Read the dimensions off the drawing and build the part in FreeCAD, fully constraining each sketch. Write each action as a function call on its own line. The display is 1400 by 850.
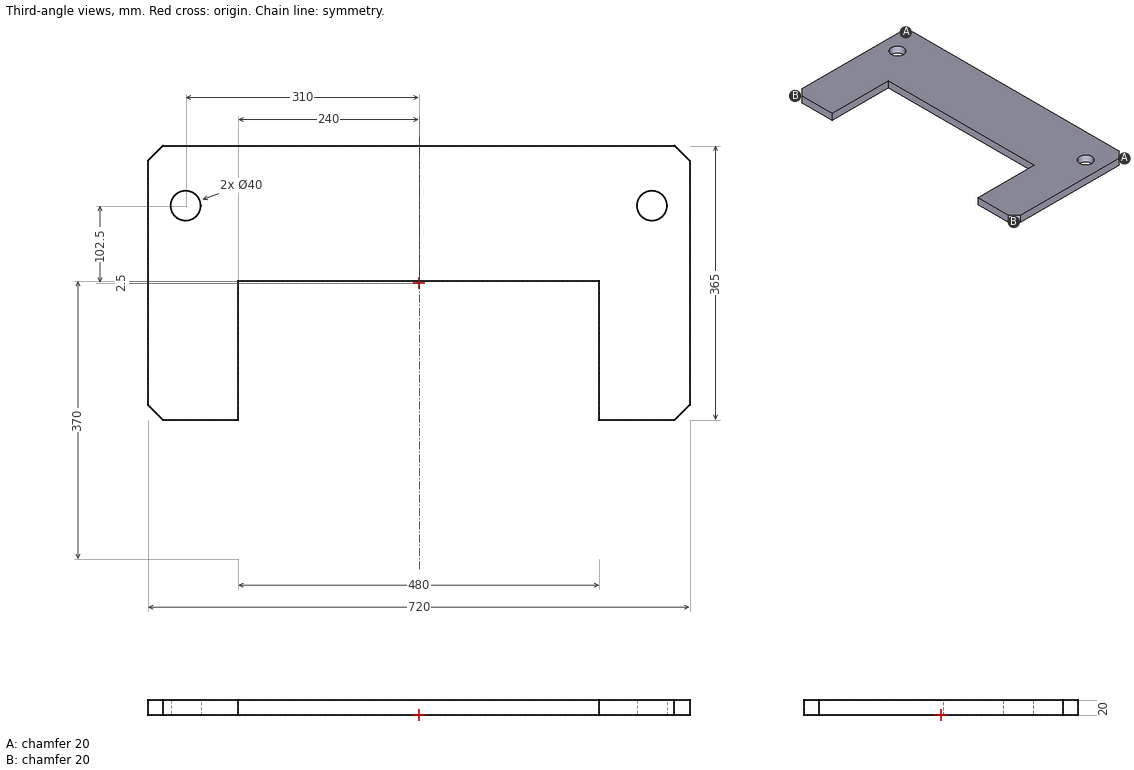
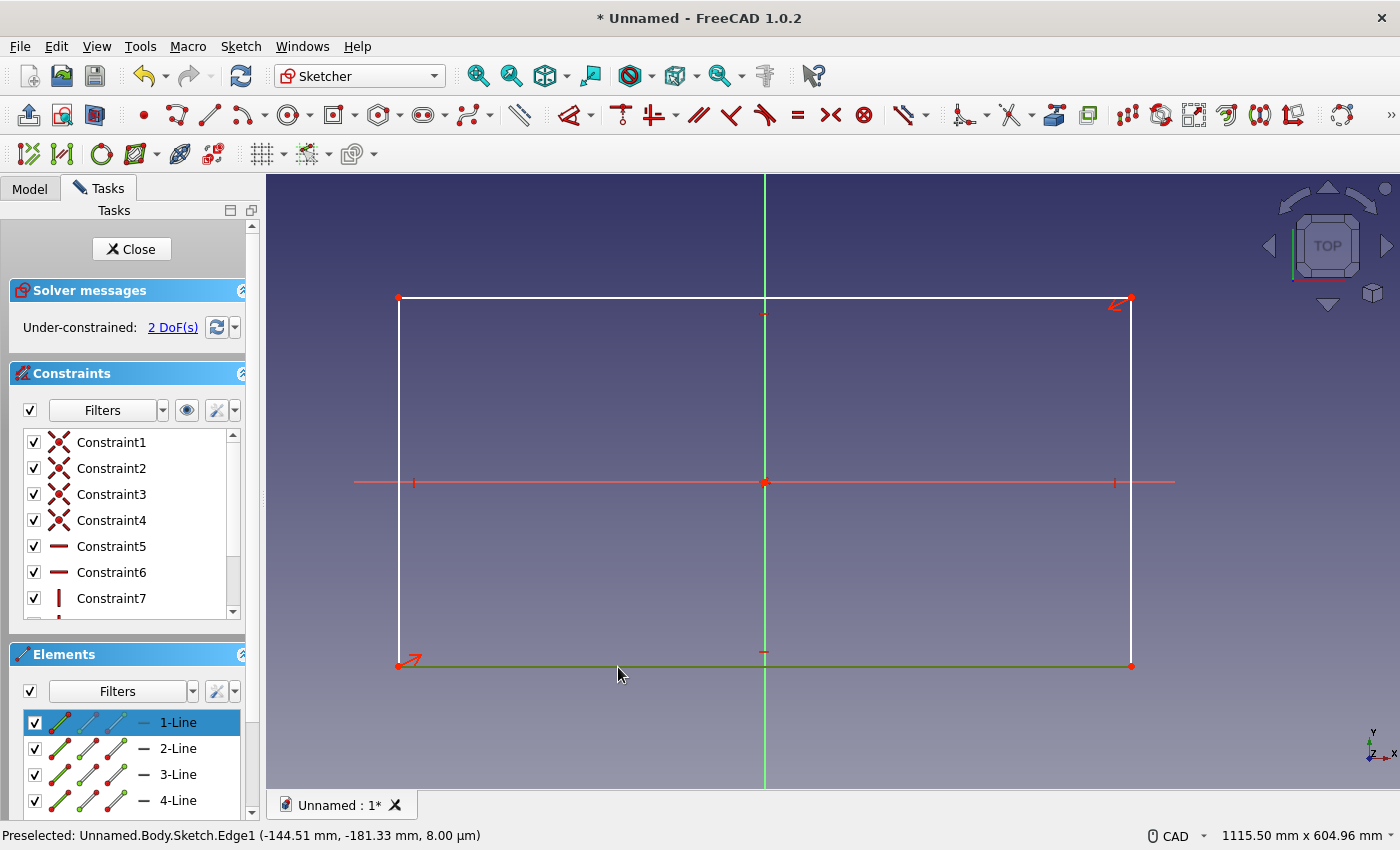
click(590, 116)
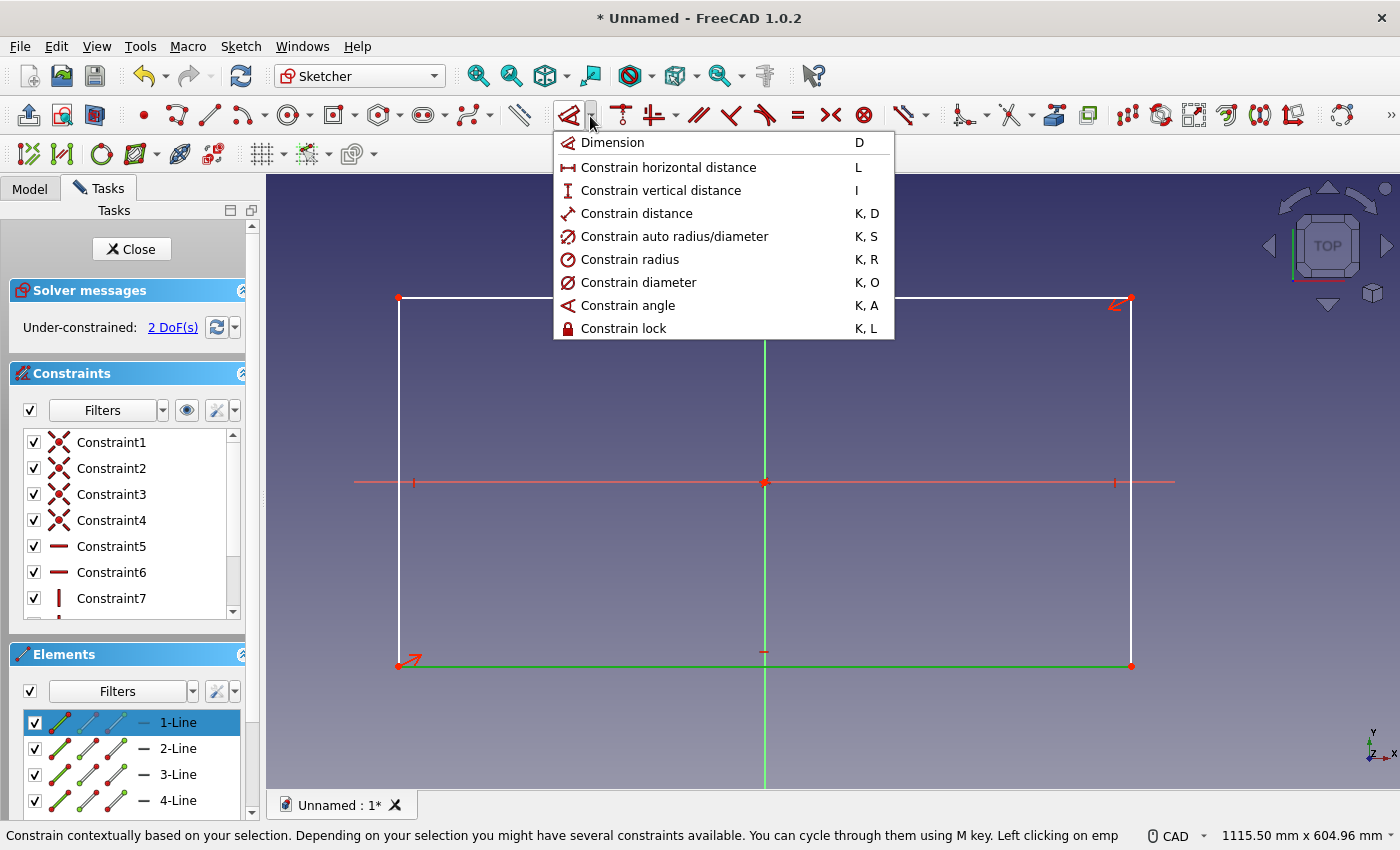
click(724, 168)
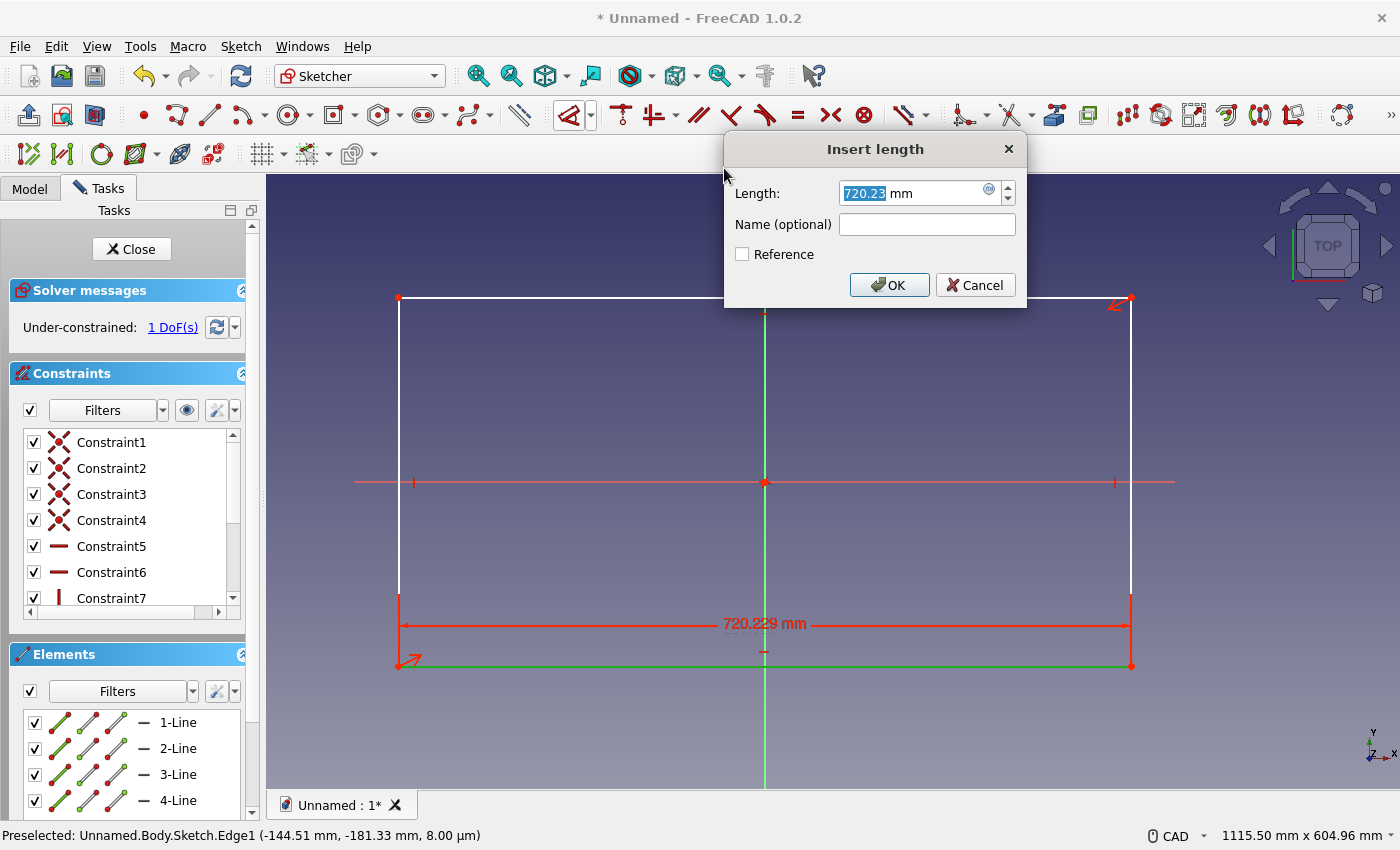
text(720)
key(Return)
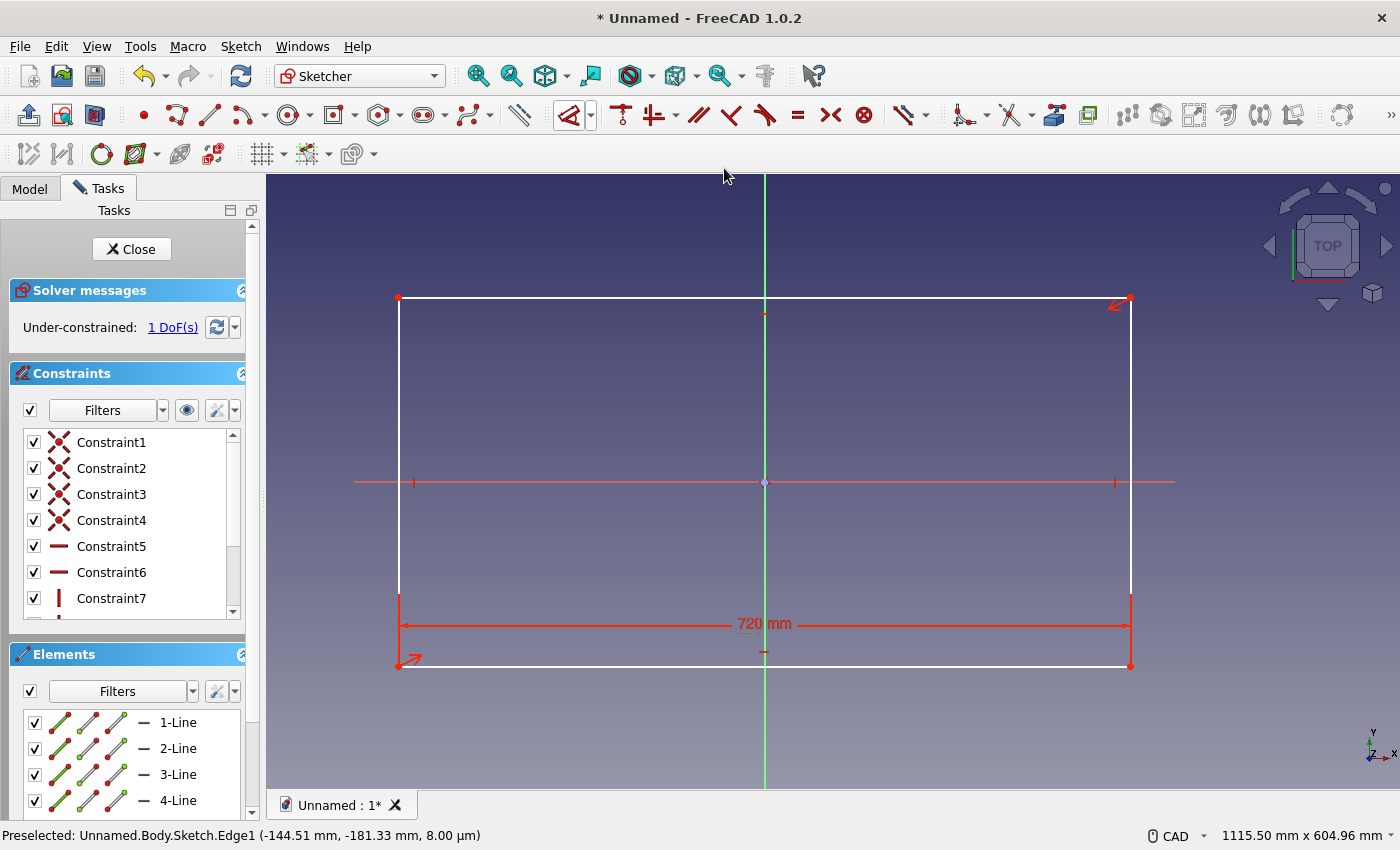
click(1131, 556)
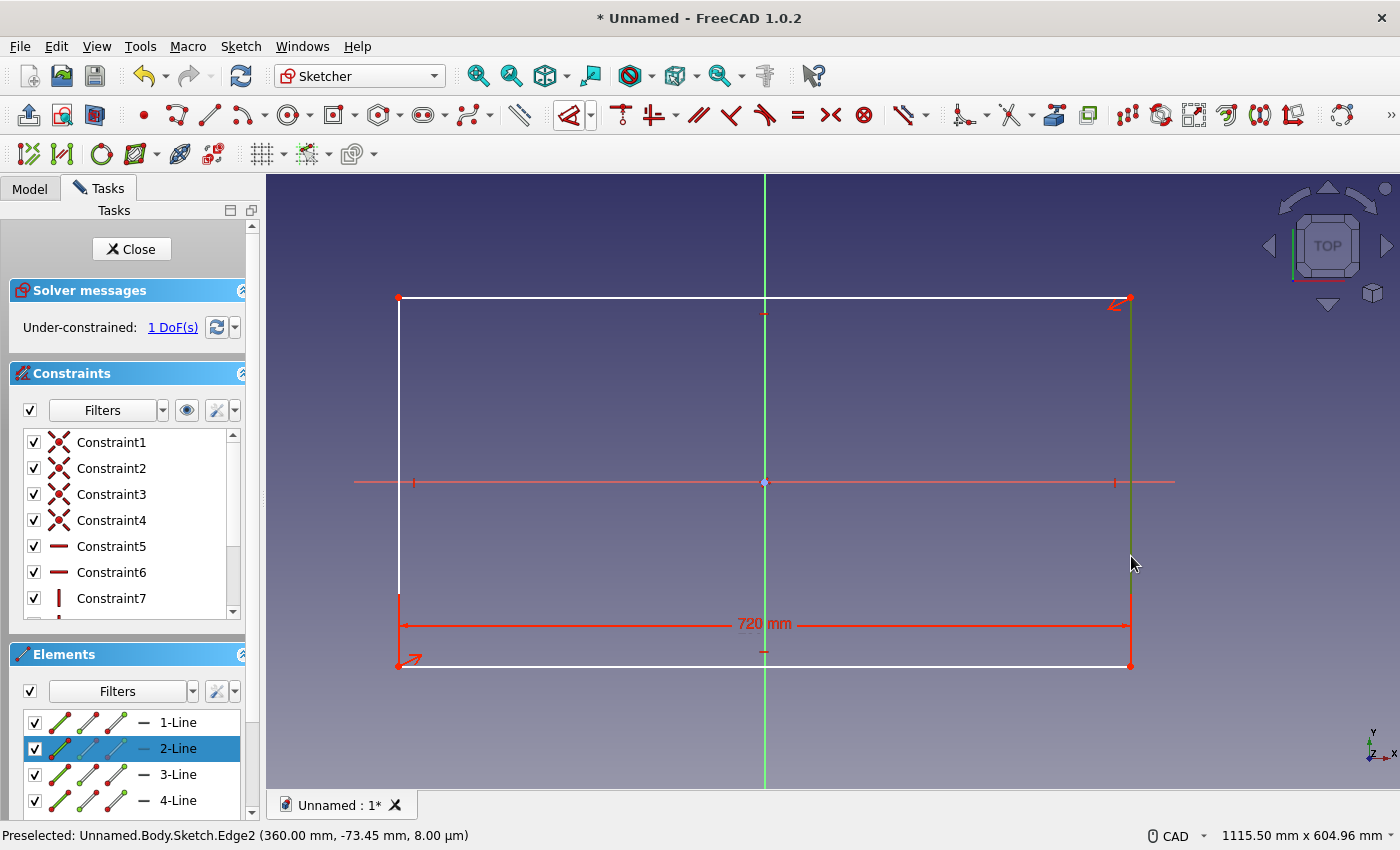
key(i)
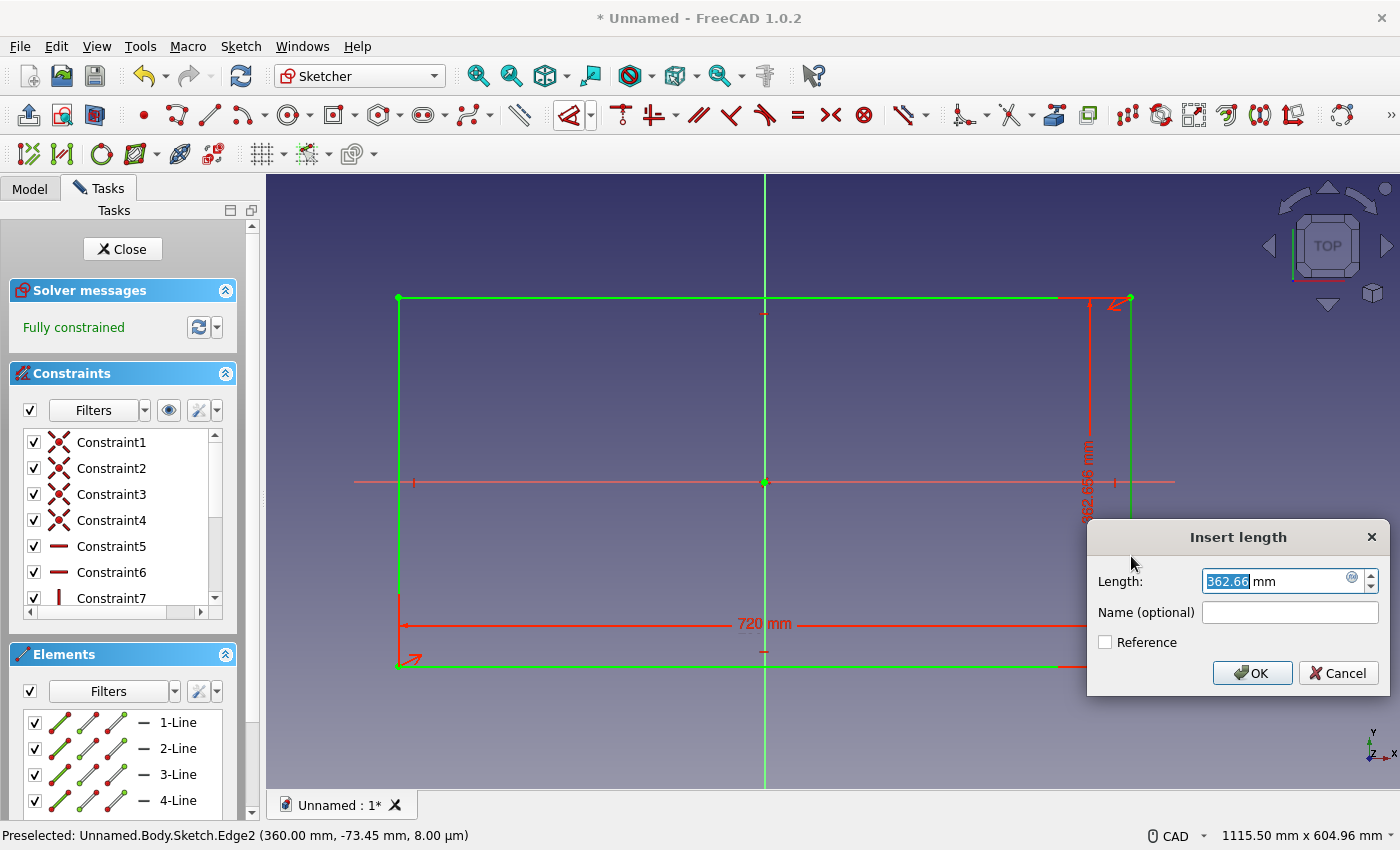
text(365)
key(Return)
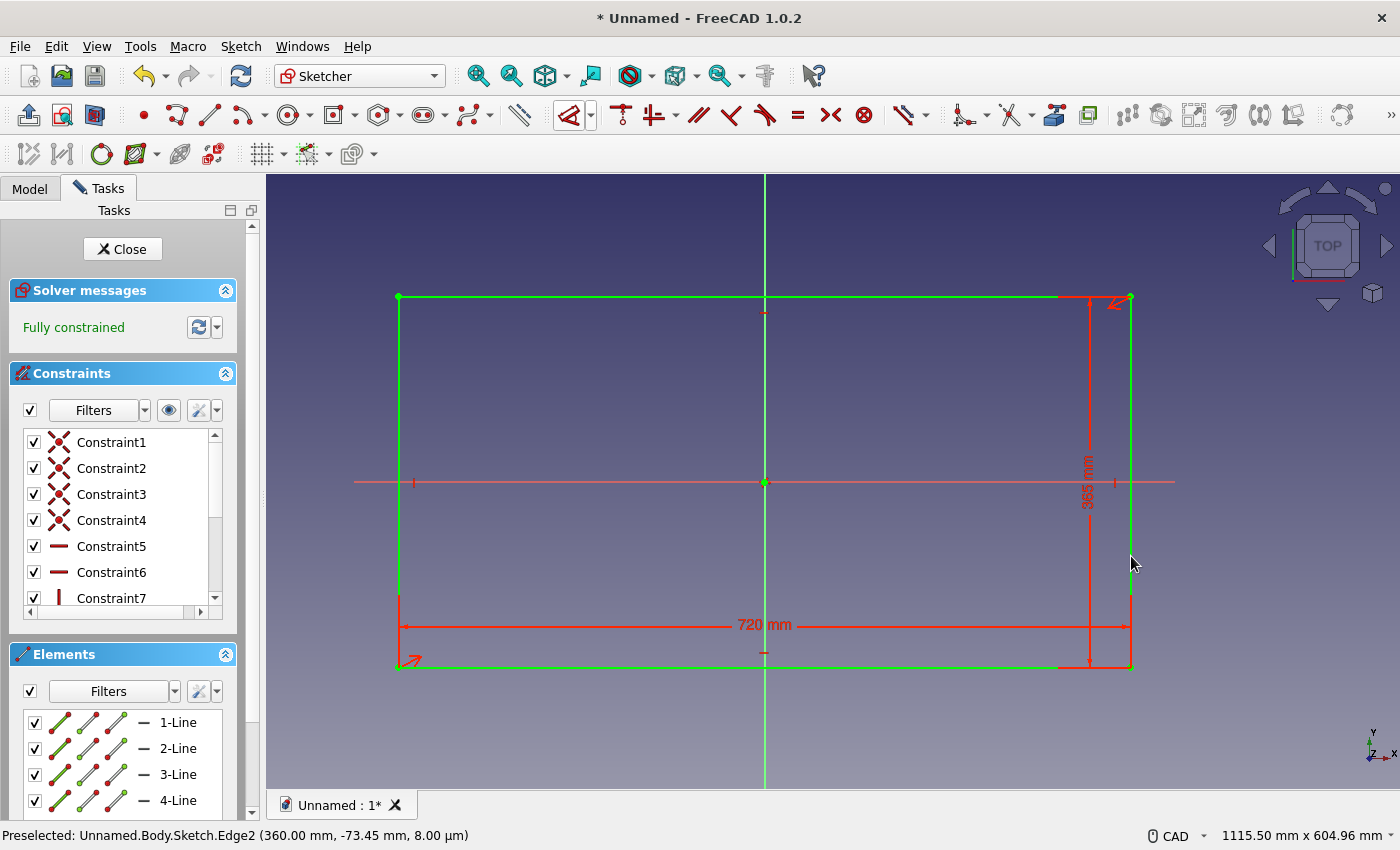
click(123, 249)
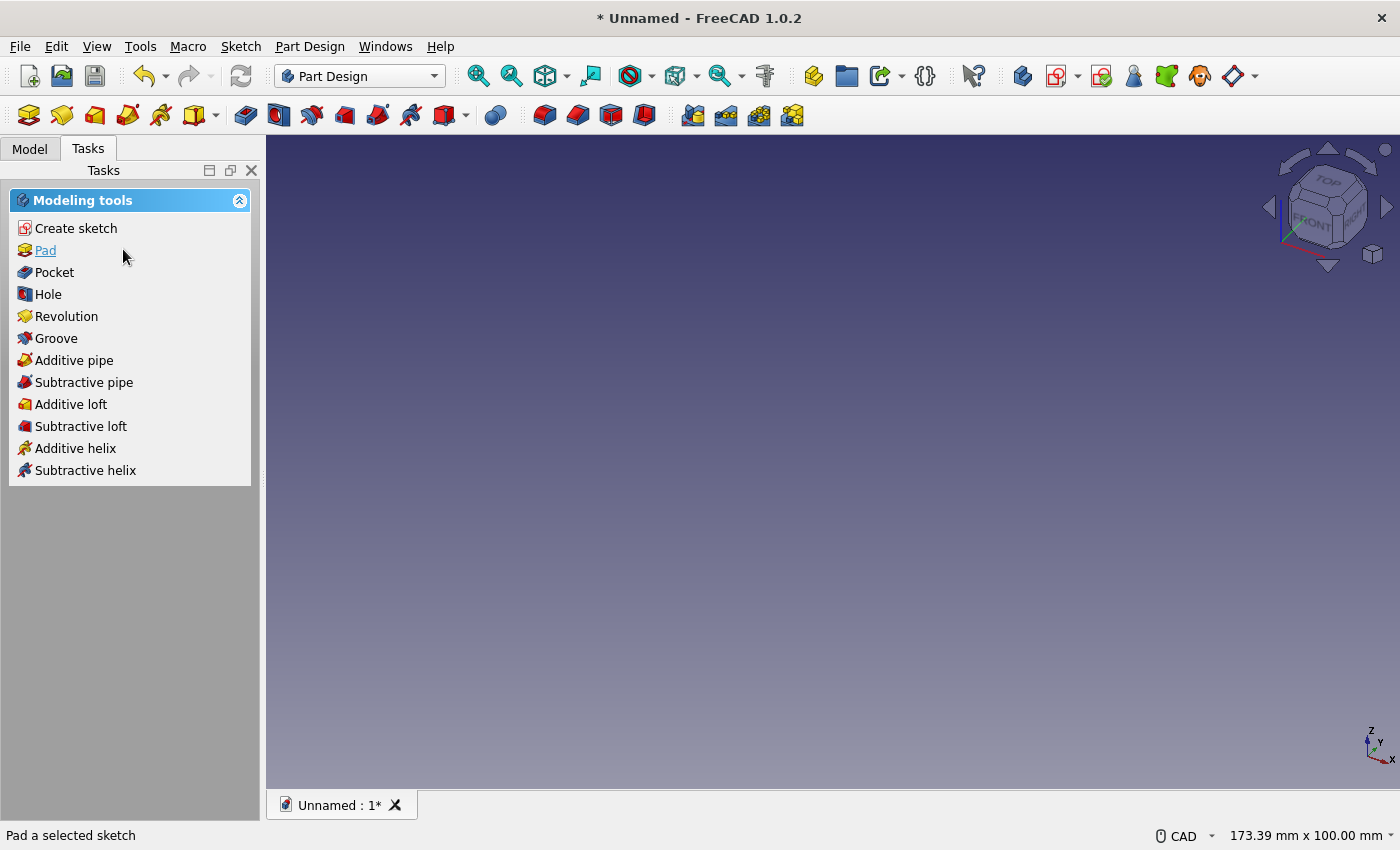
click(29, 116)